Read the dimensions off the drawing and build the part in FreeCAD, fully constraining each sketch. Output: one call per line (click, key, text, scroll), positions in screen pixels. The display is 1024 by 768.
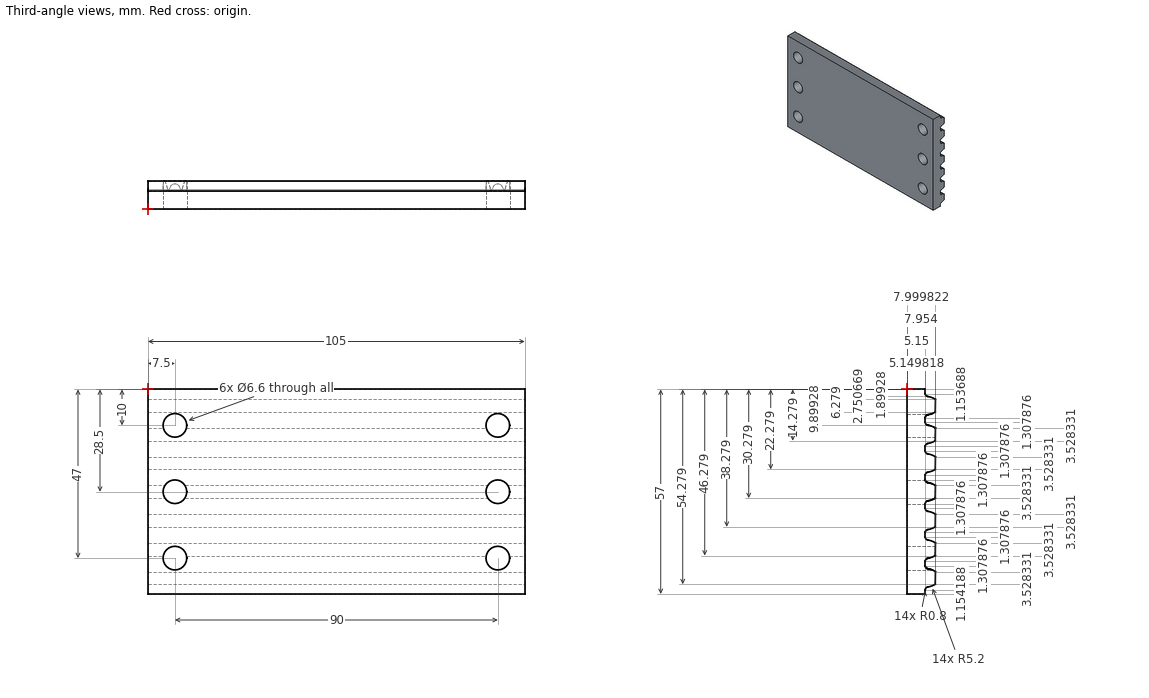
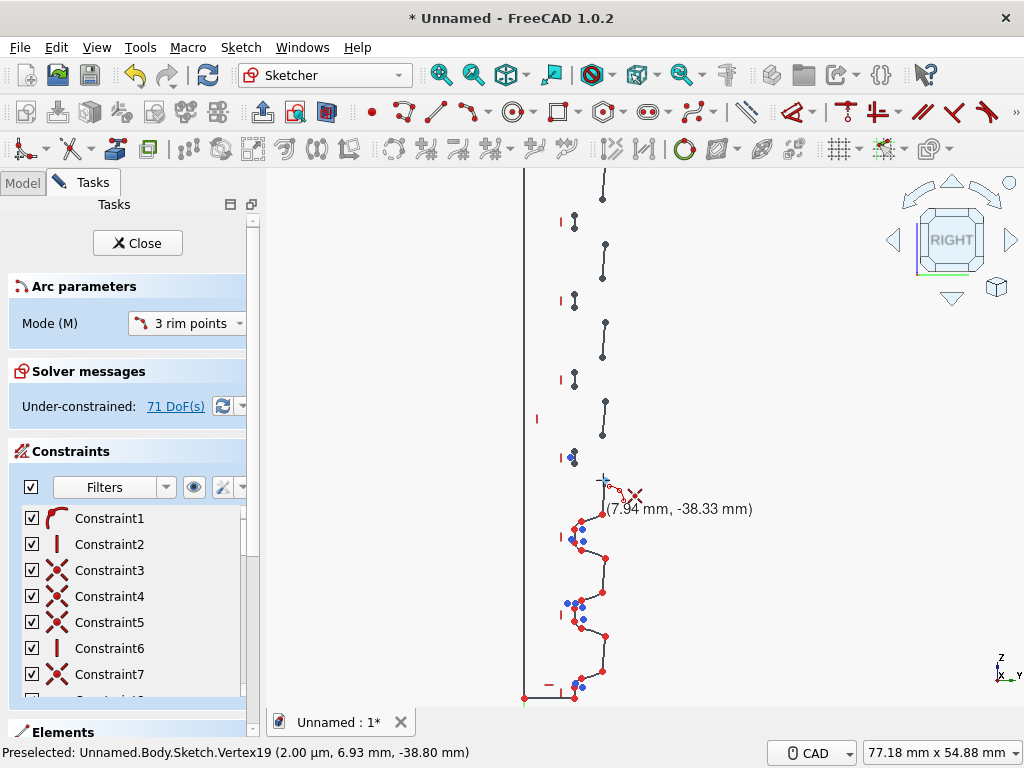
click(605, 480)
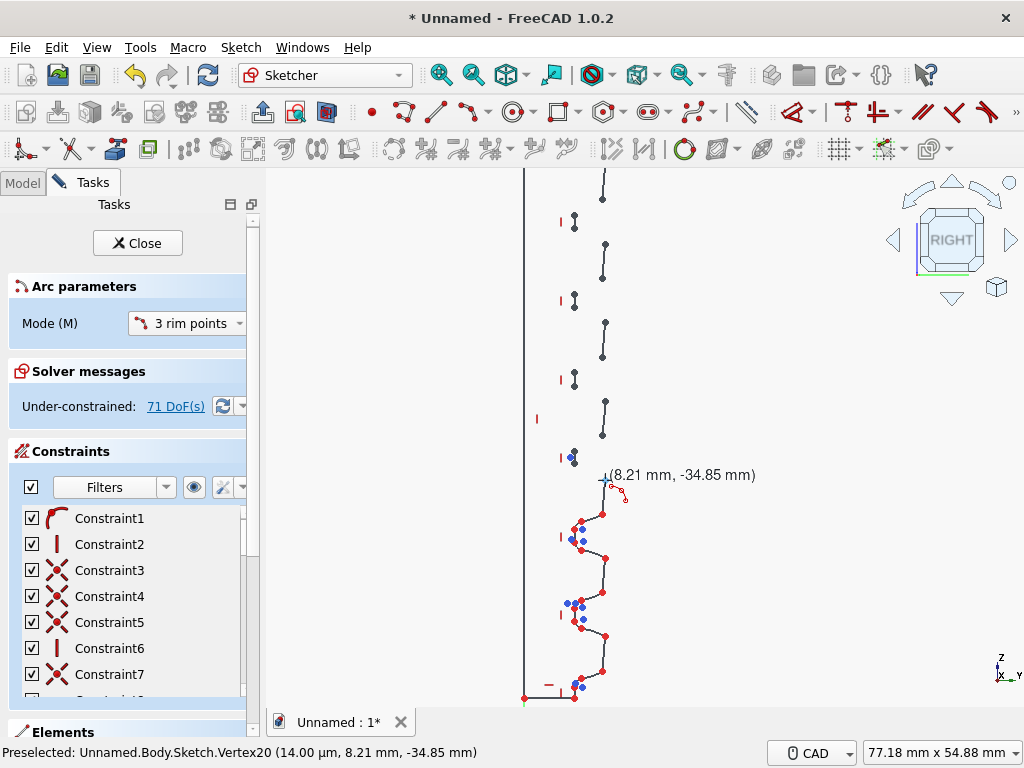
scroll(582, 471, up, 5)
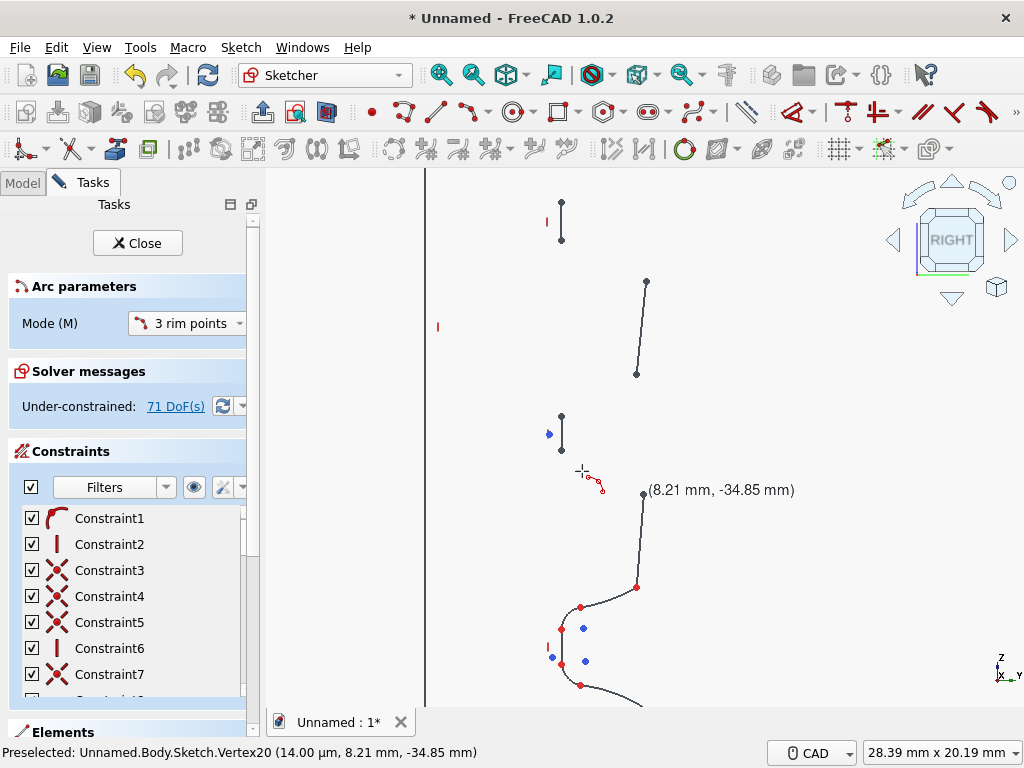
click(581, 471)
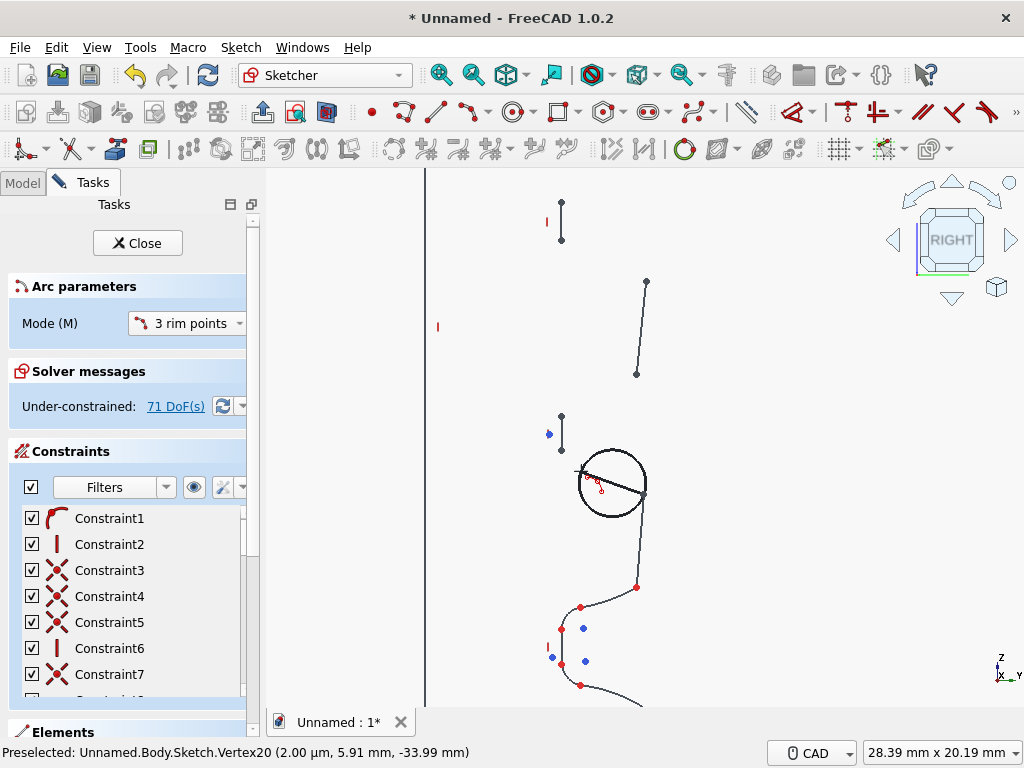
scroll(611, 478, up, 8)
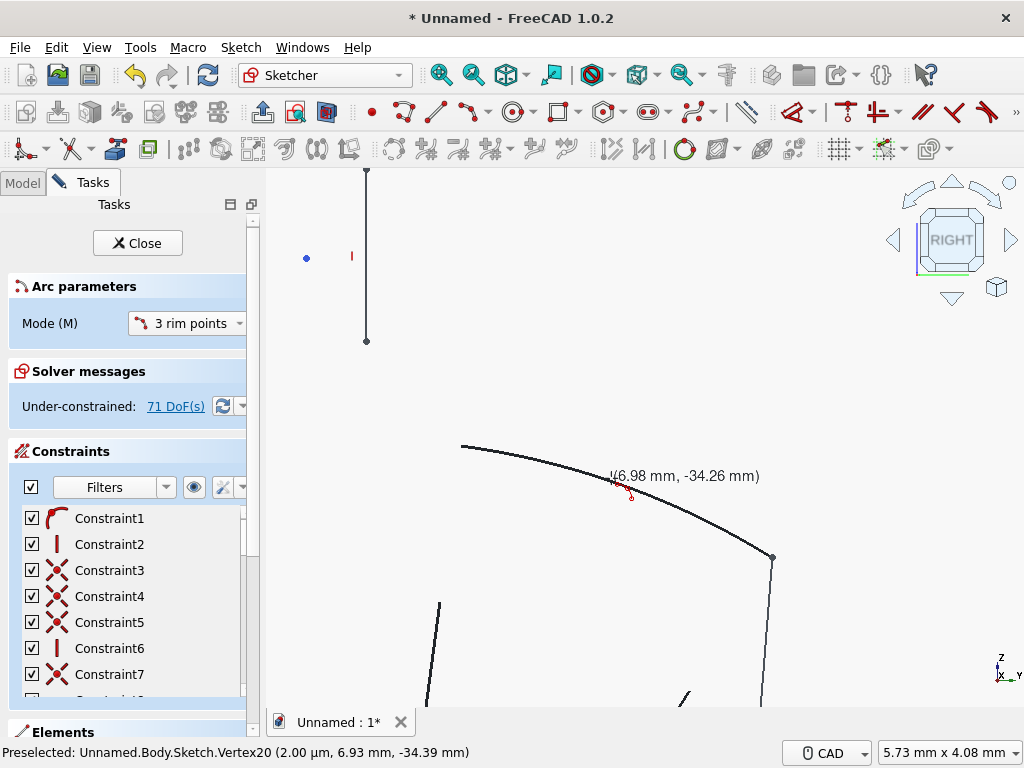
click(608, 476)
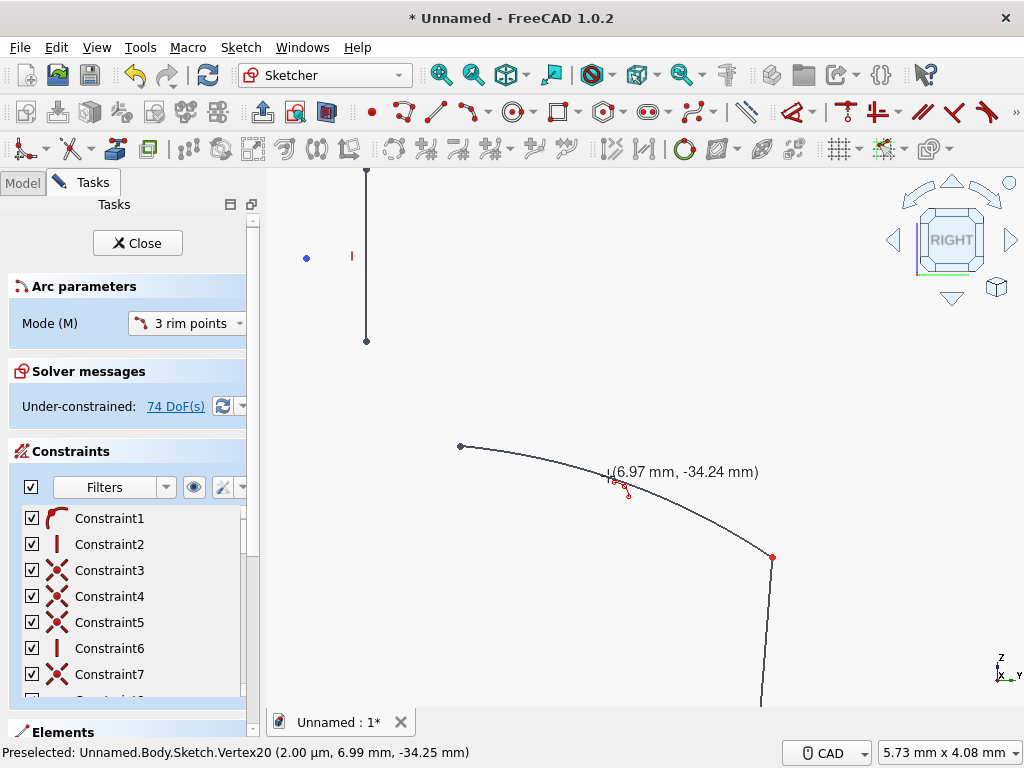
scroll(595, 475, down, 15)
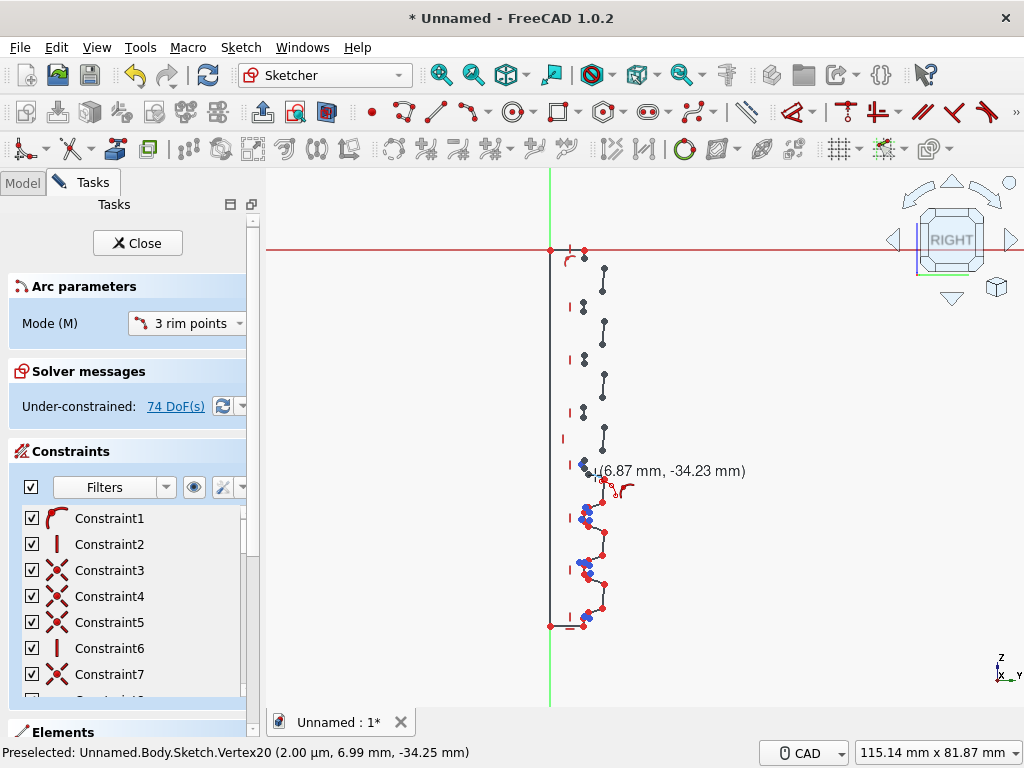
scroll(589, 474, up, 7)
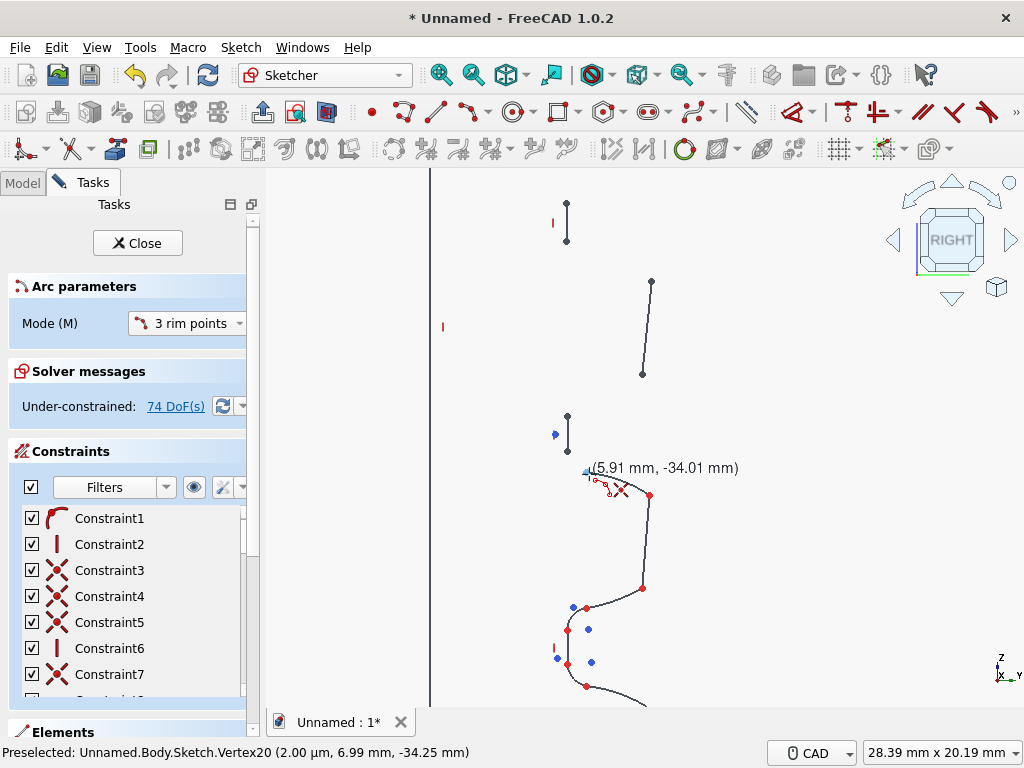
click(587, 473)
click(568, 452)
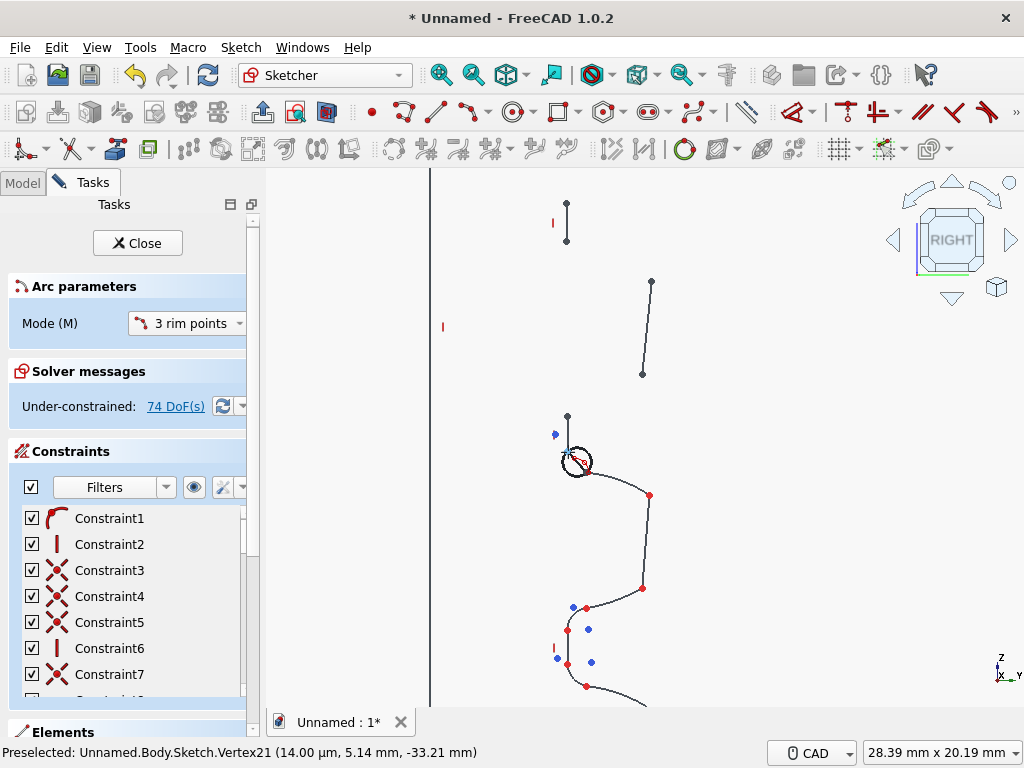
scroll(573, 464, up, 6)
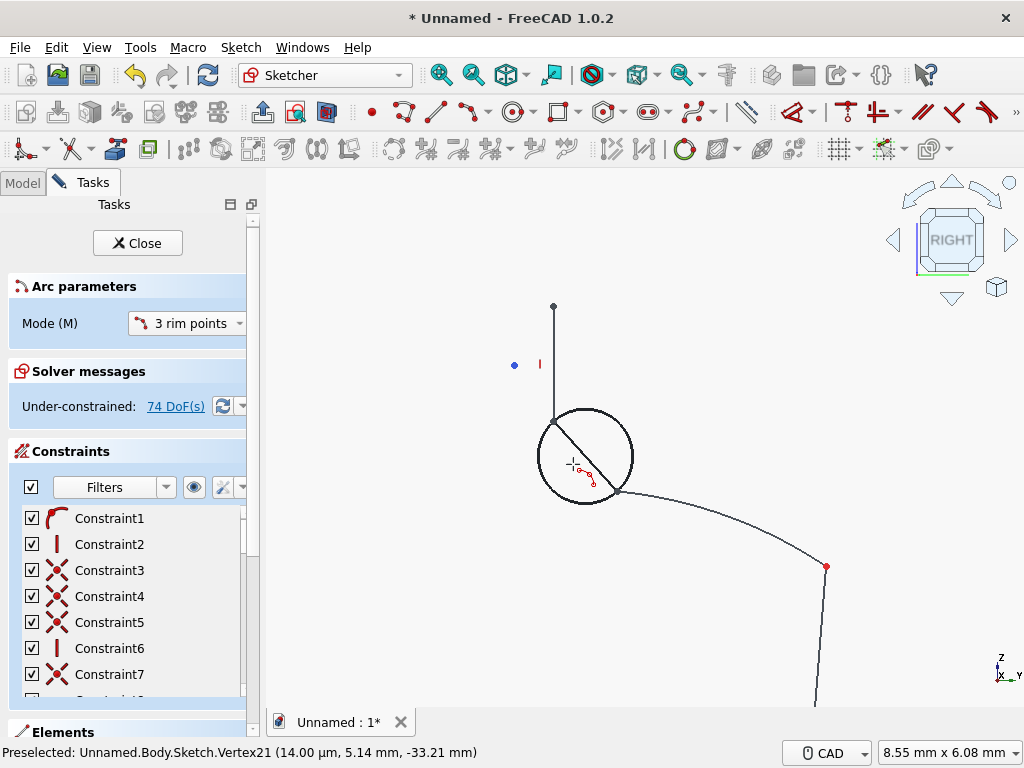
click(572, 463)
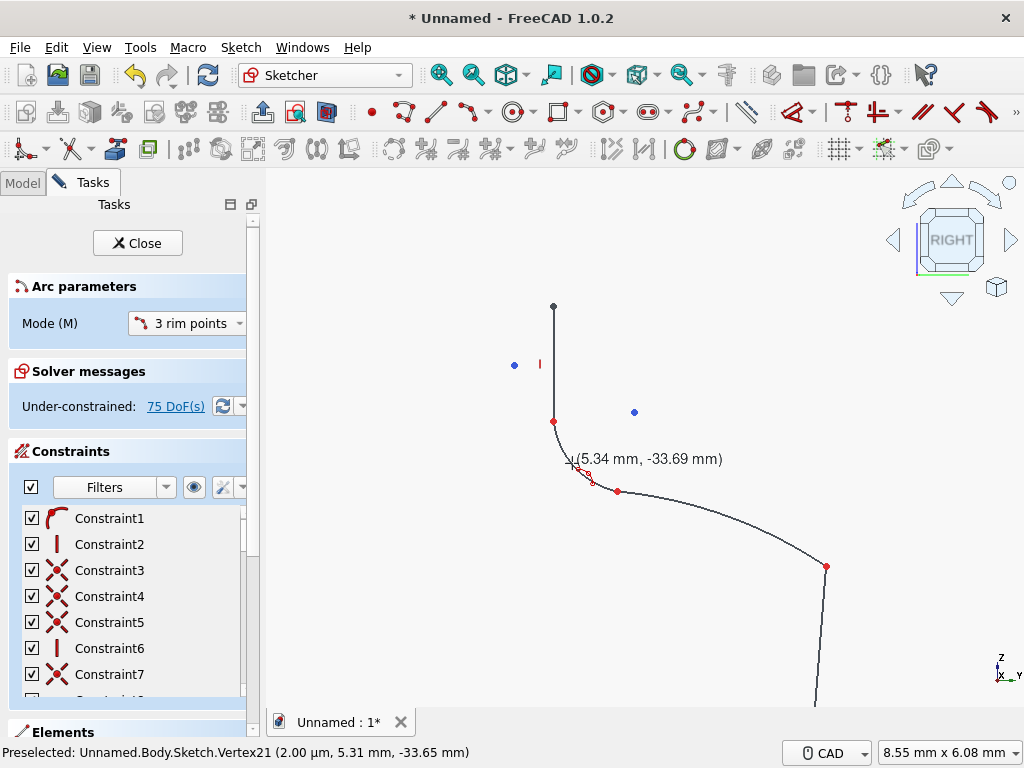
scroll(586, 472, down, 13)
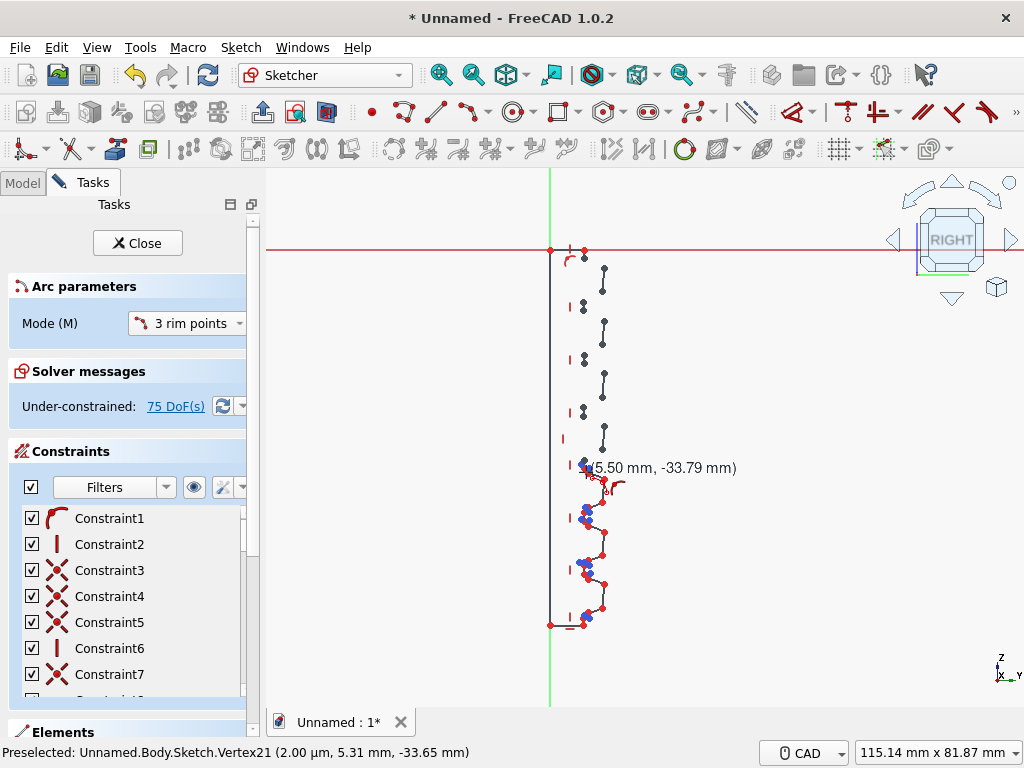
scroll(584, 460, up, 7)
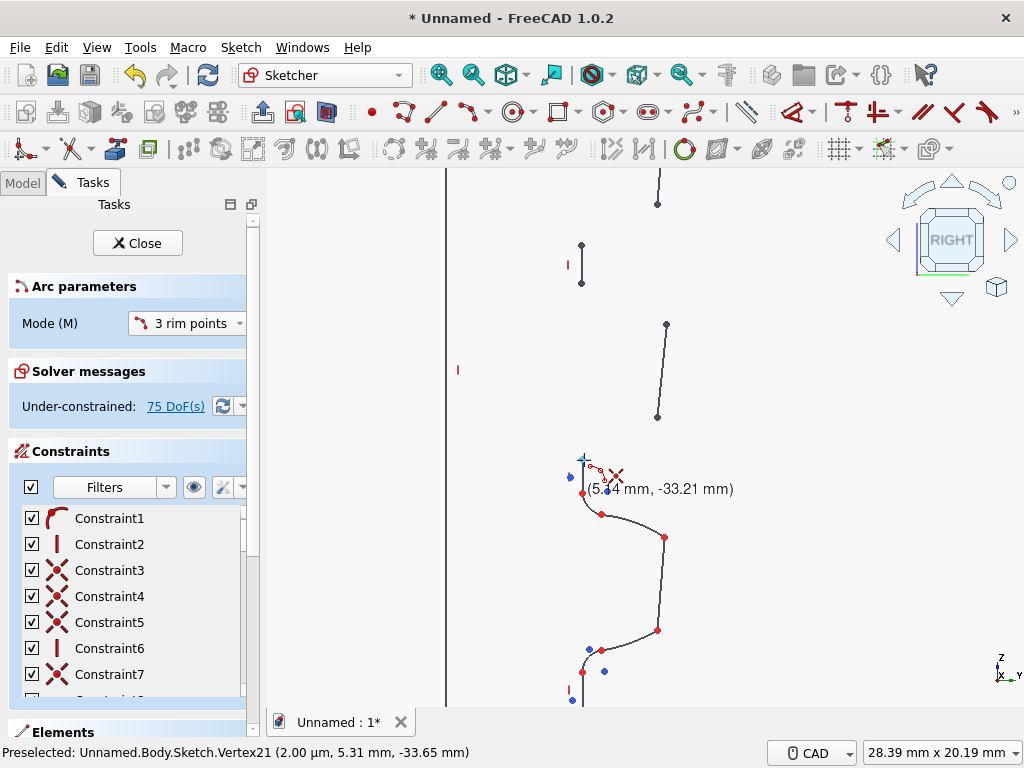
click(583, 459)
click(602, 436)